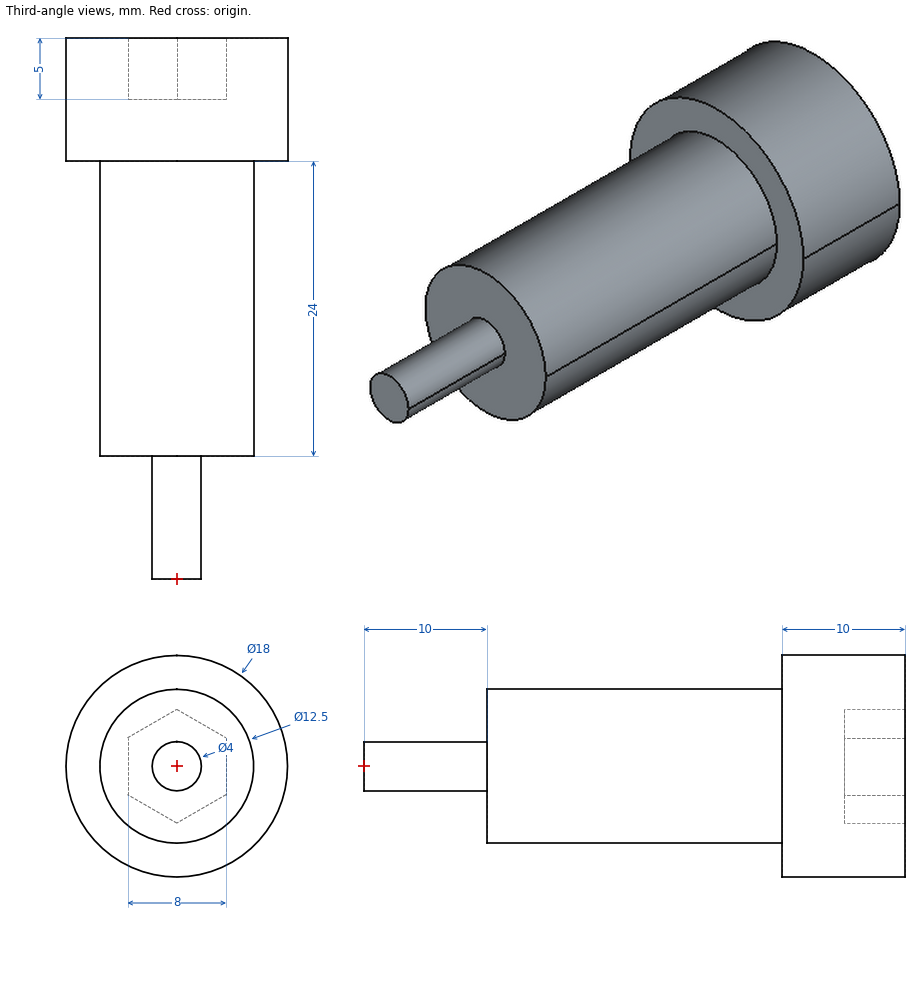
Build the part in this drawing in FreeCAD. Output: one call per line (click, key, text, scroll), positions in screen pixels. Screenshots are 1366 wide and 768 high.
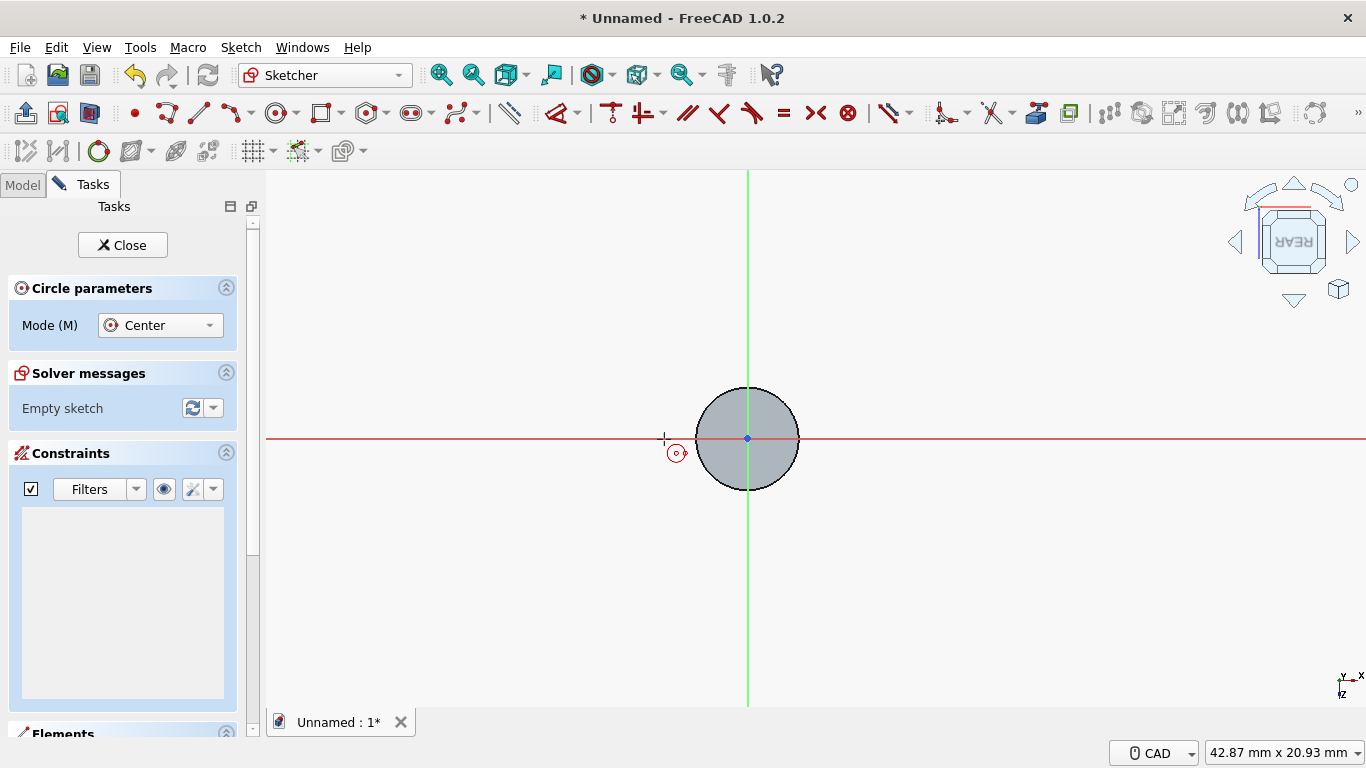
click(748, 439)
move(861, 326)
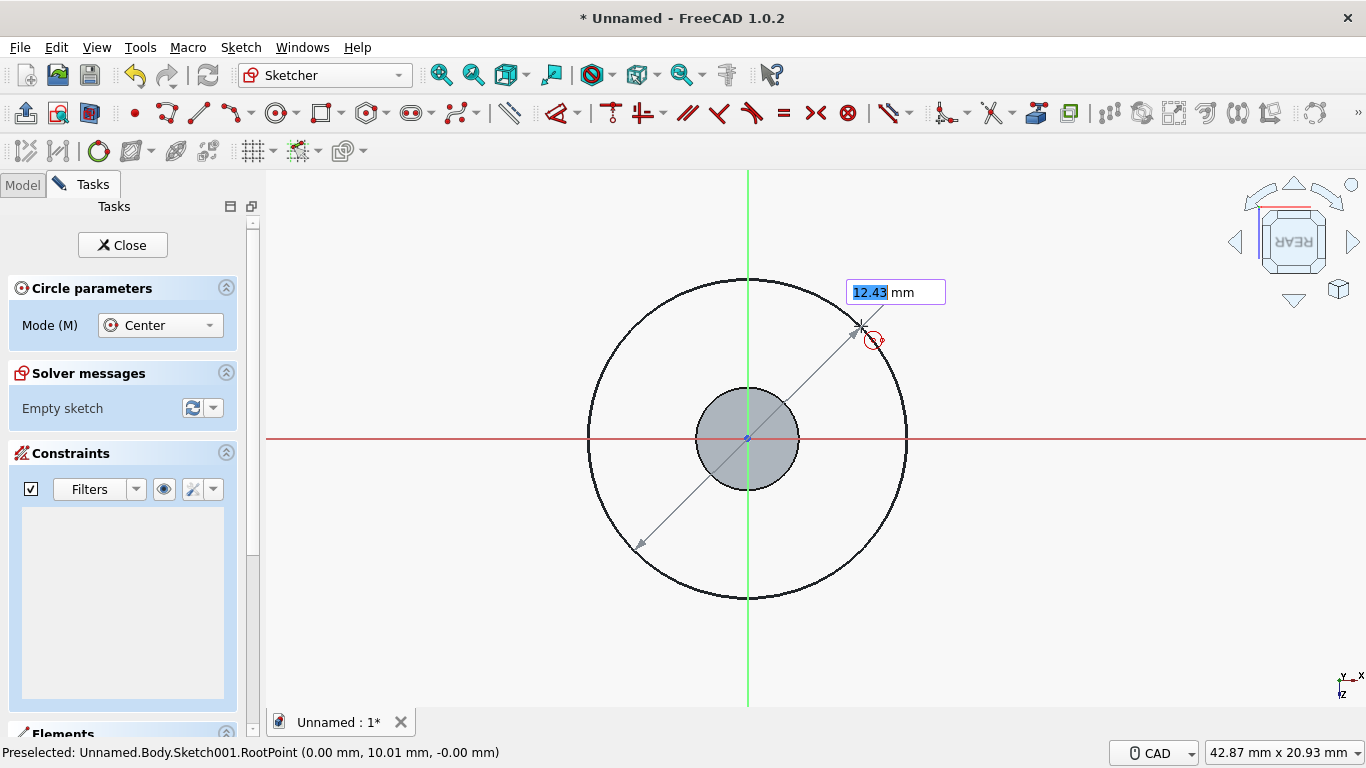
text(12.5)
key(Return)
key(Escape)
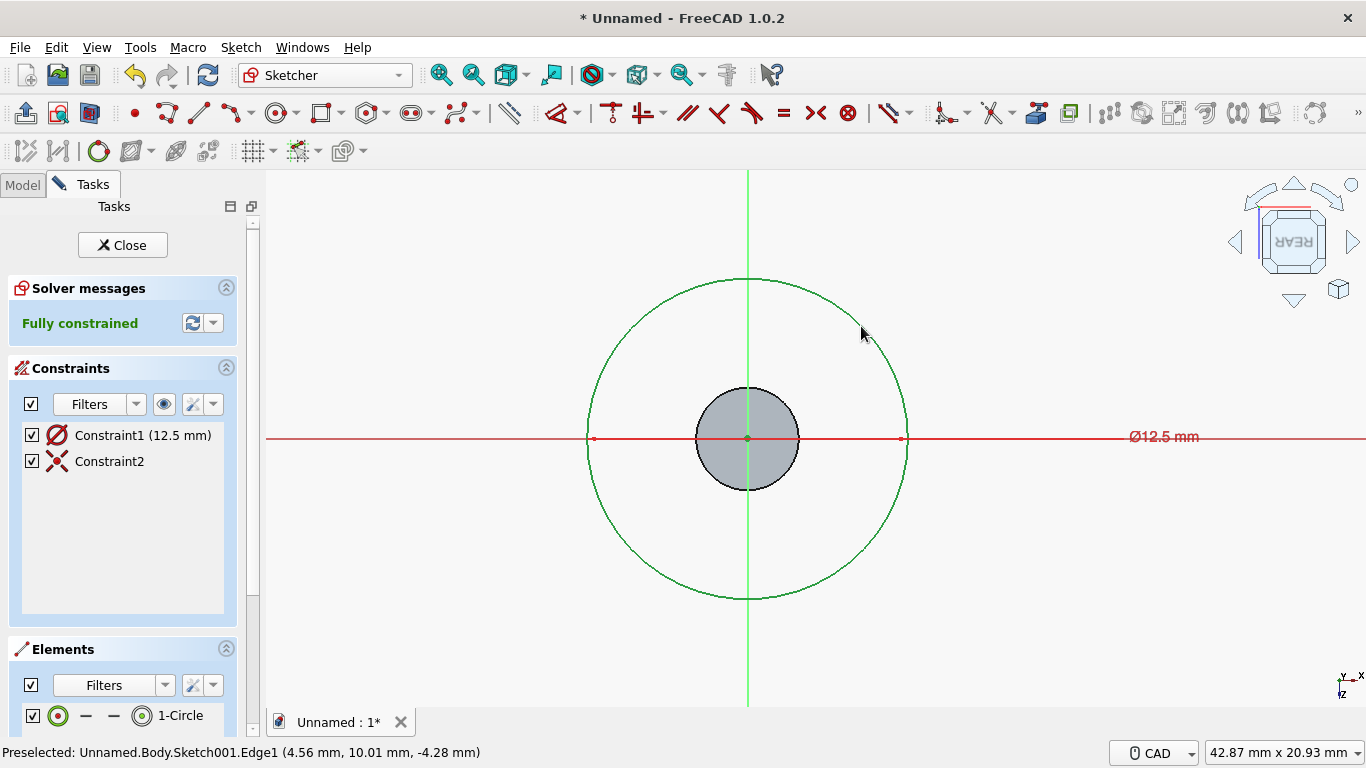
click(123, 245)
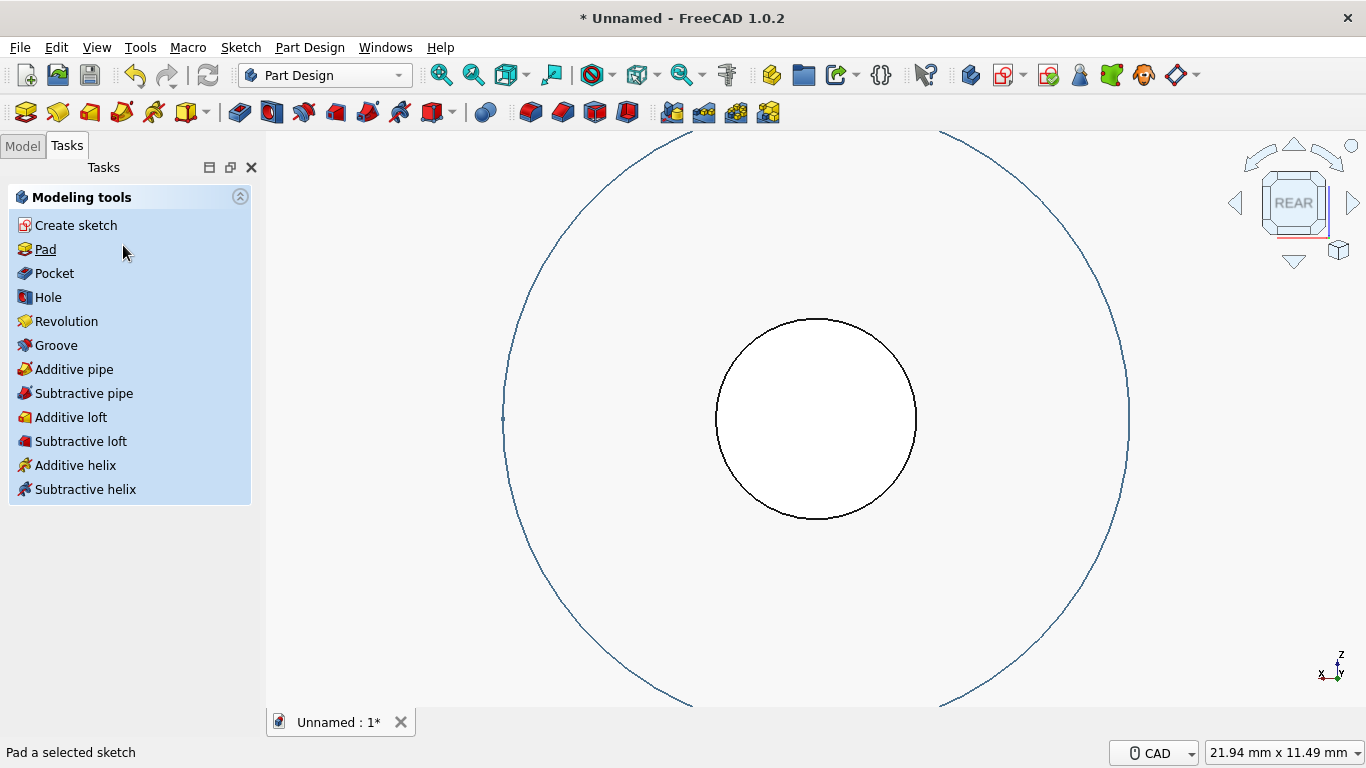
click(26, 112)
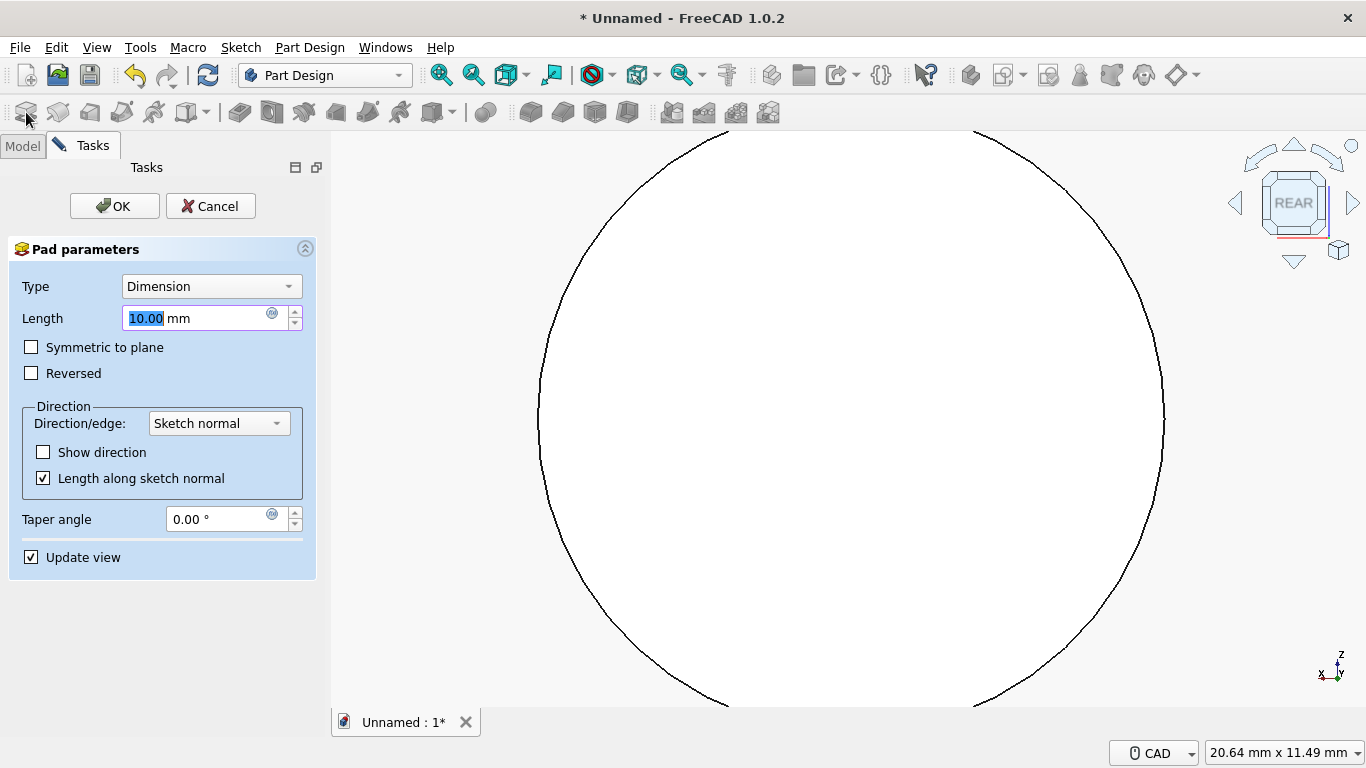
text(24)
key(Tab)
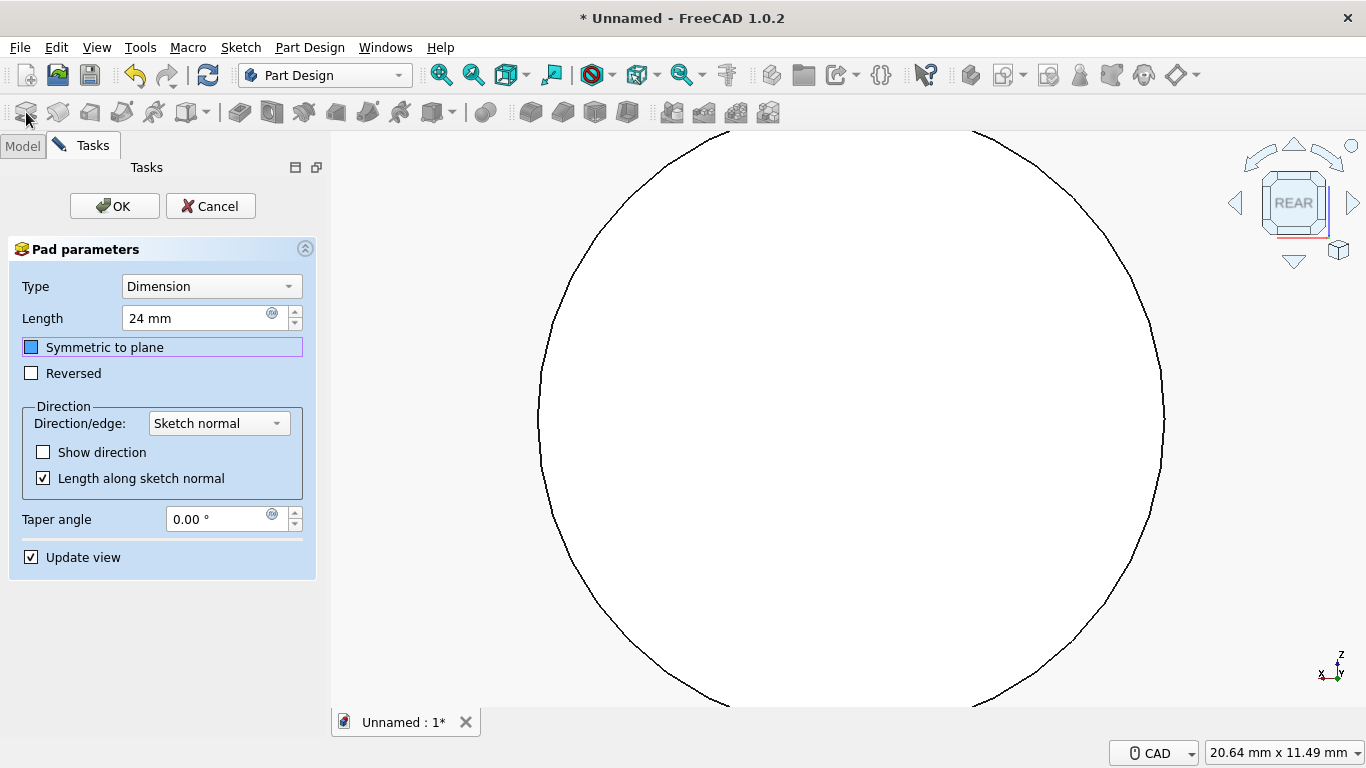
click(115, 206)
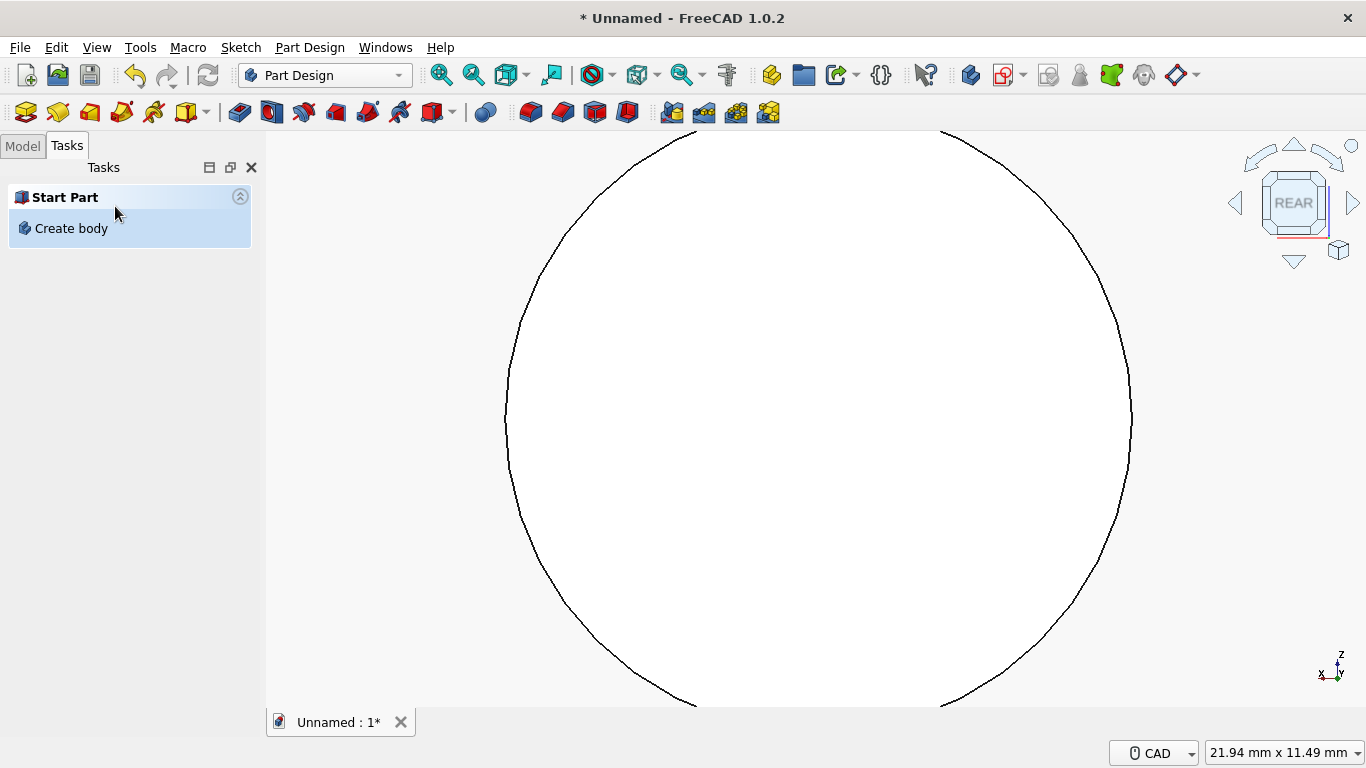
key(v)
key(f)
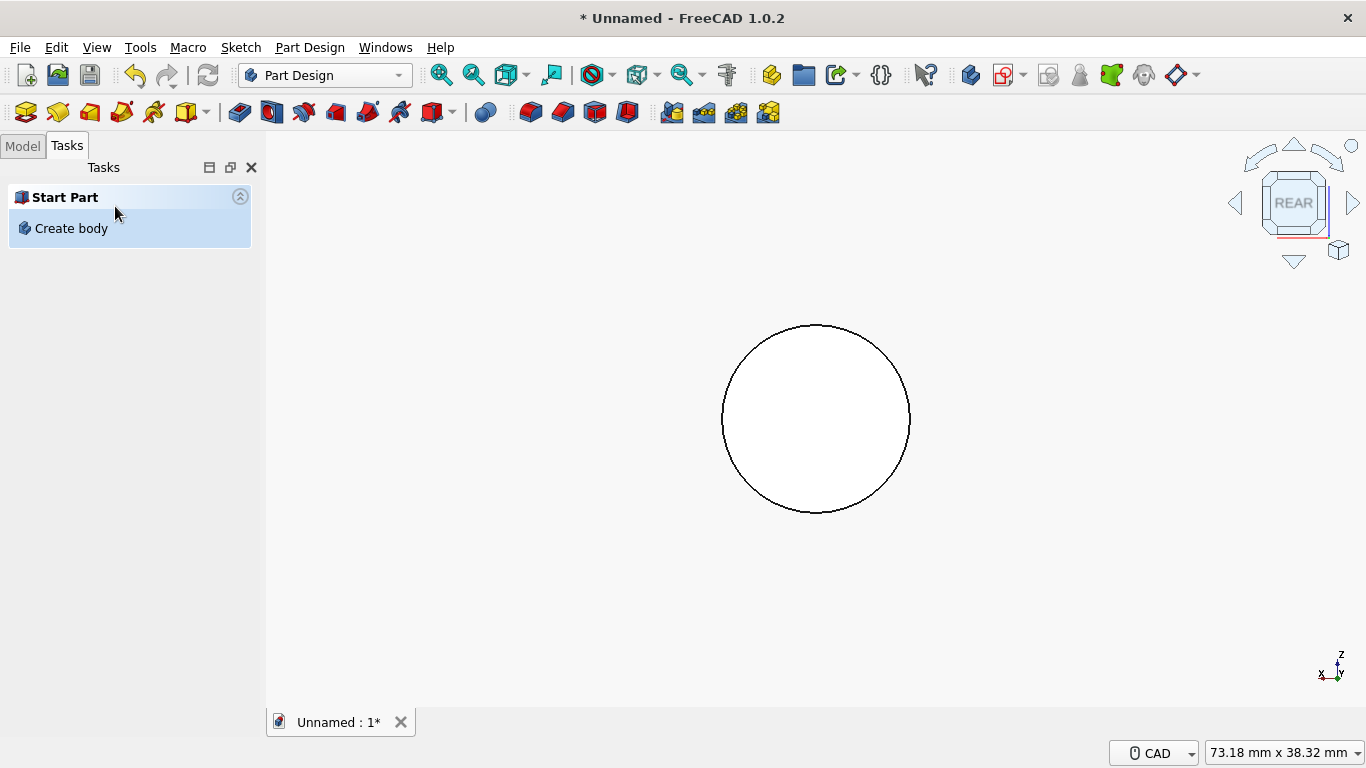
click(816, 418)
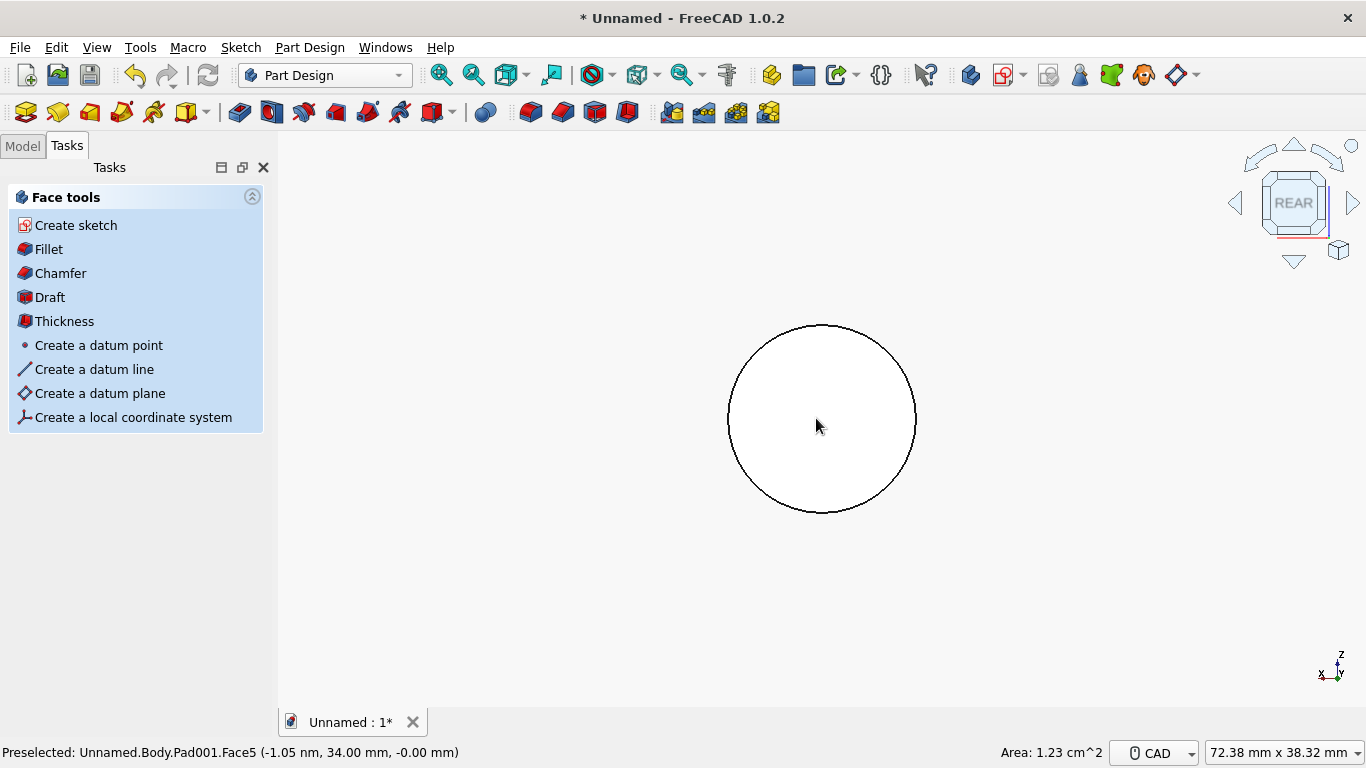
click(1004, 76)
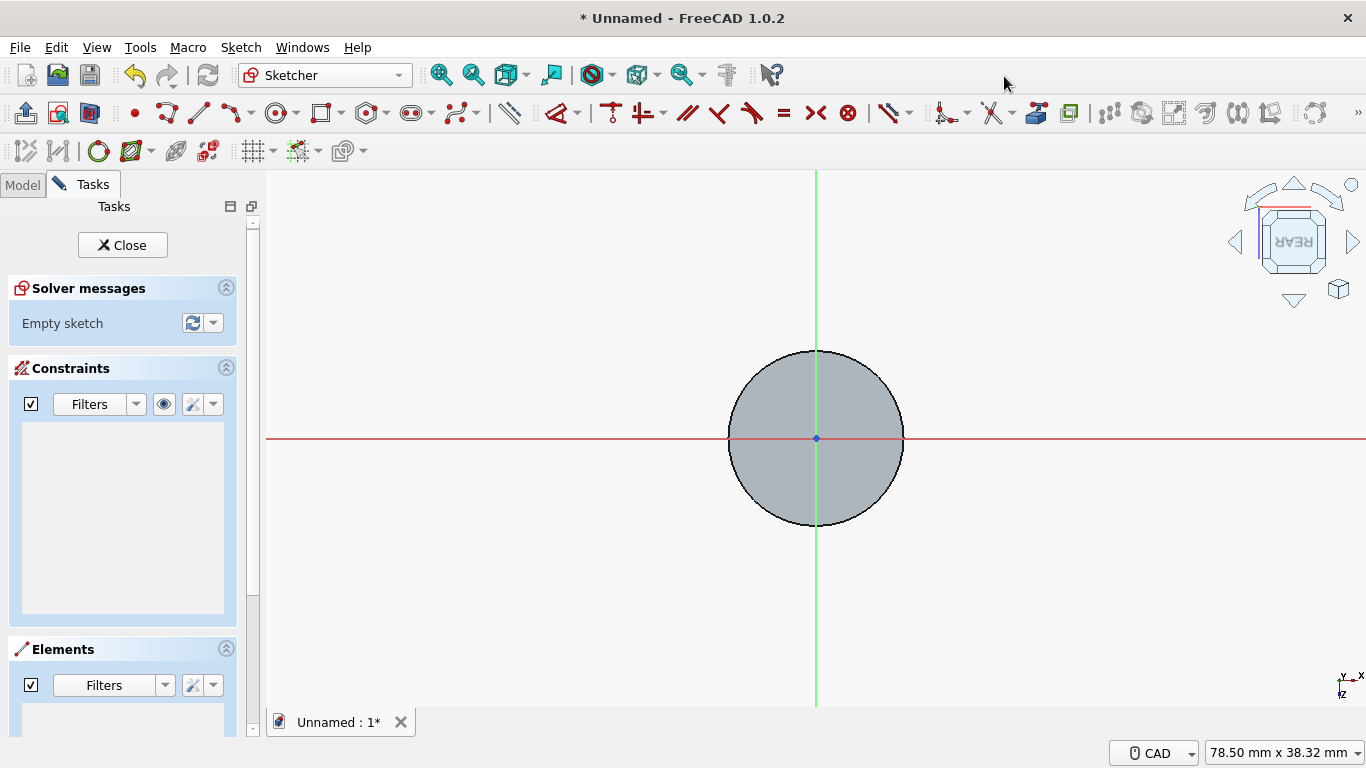
key(g)
key(c)